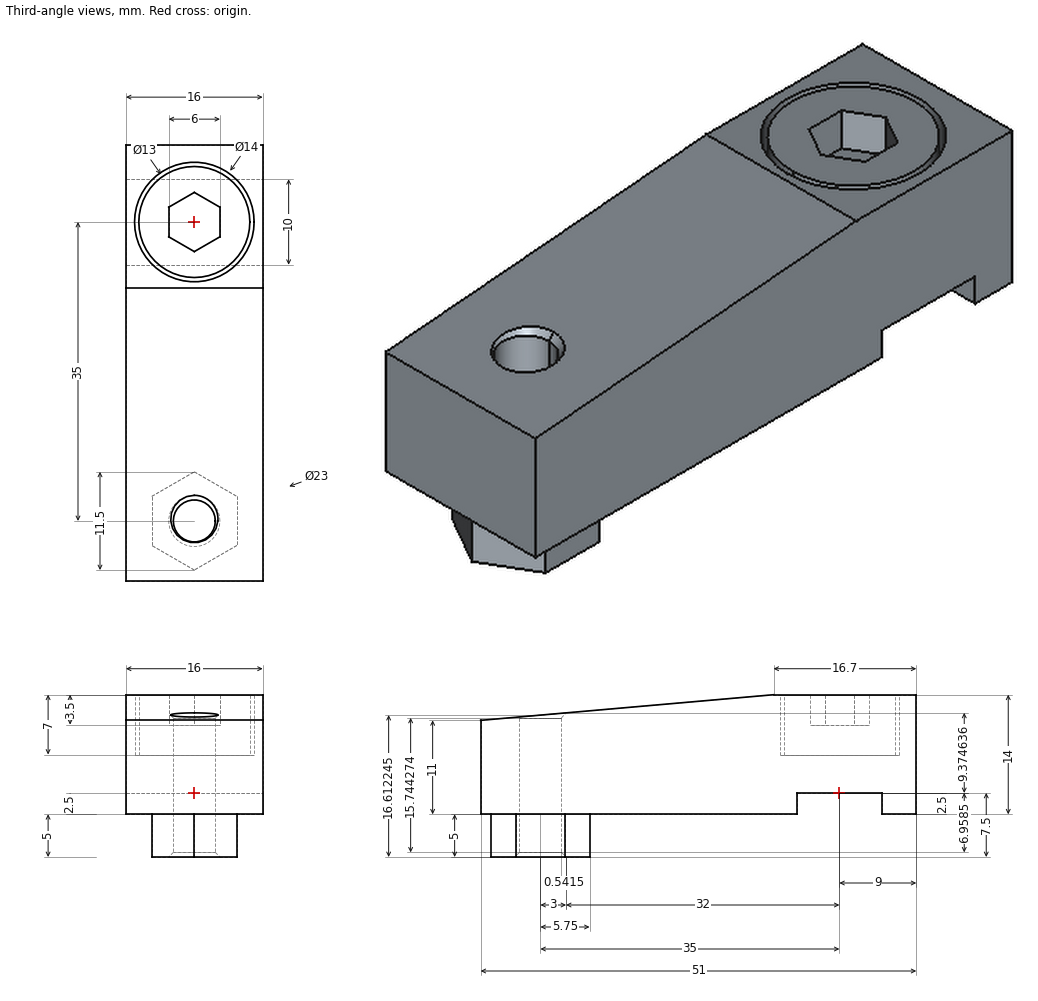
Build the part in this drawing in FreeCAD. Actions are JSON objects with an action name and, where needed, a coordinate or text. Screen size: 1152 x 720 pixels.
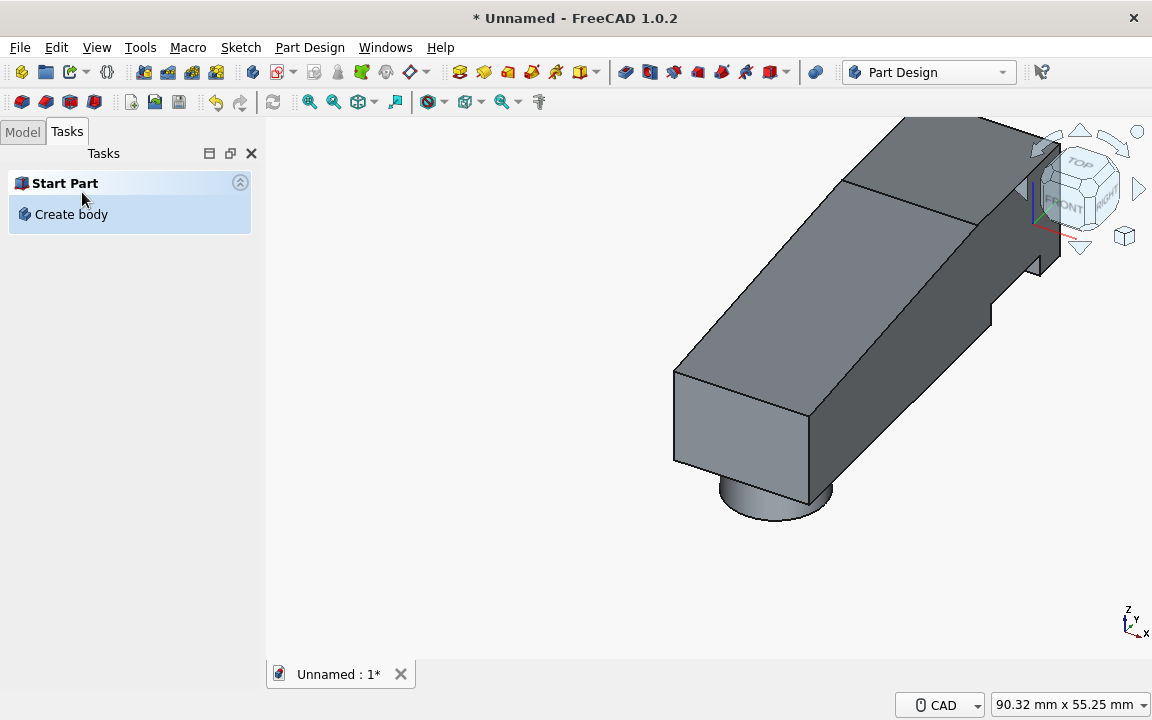
{"action": "left_click", "coordinate": [310, 102]}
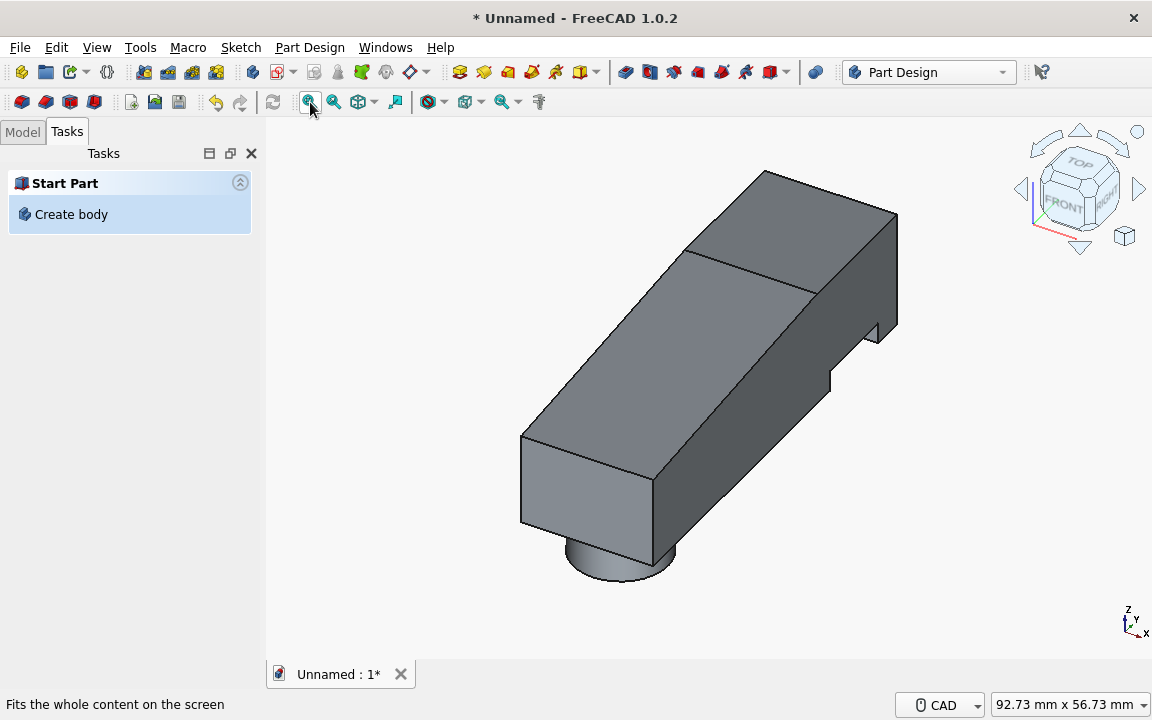
{"action": "key", "text": "5"}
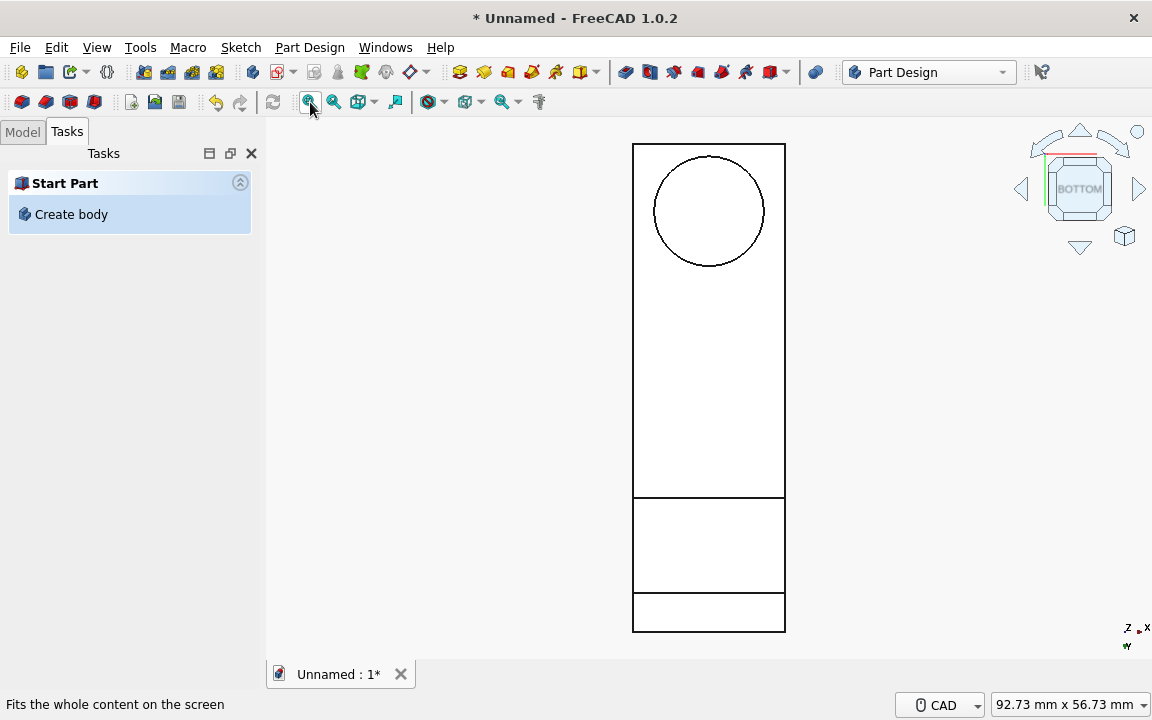
{"action": "left_click", "coordinate": [709, 210]}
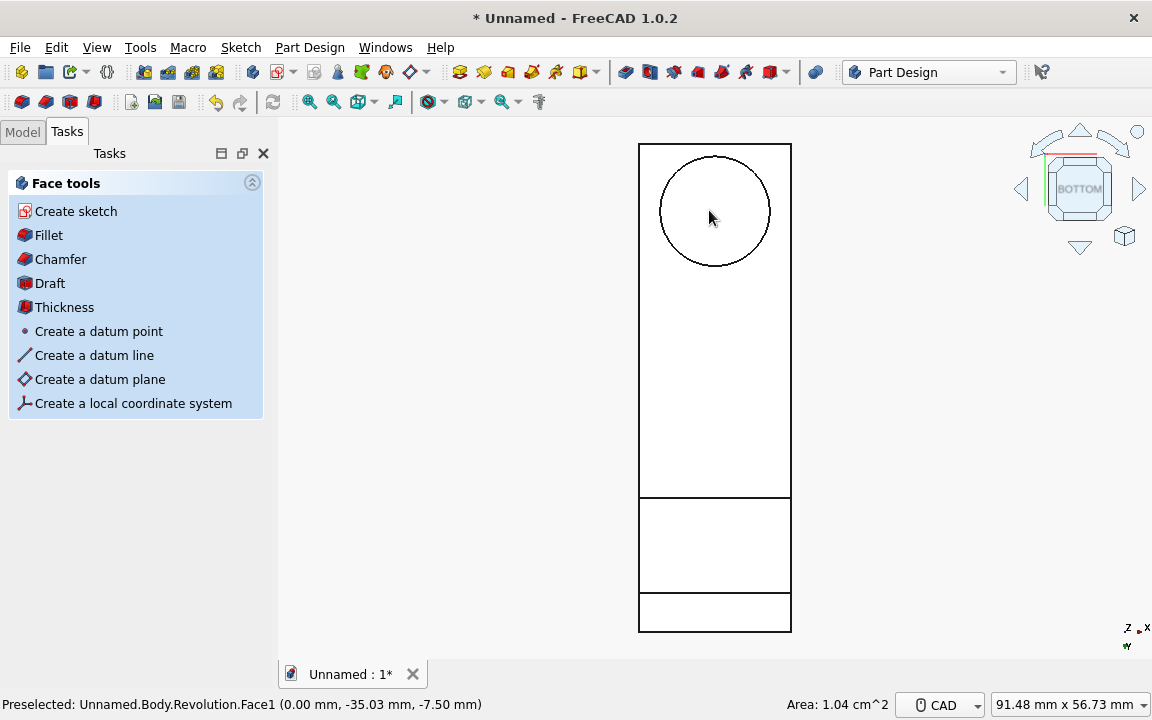
{"action": "left_click", "coordinate": [278, 72]}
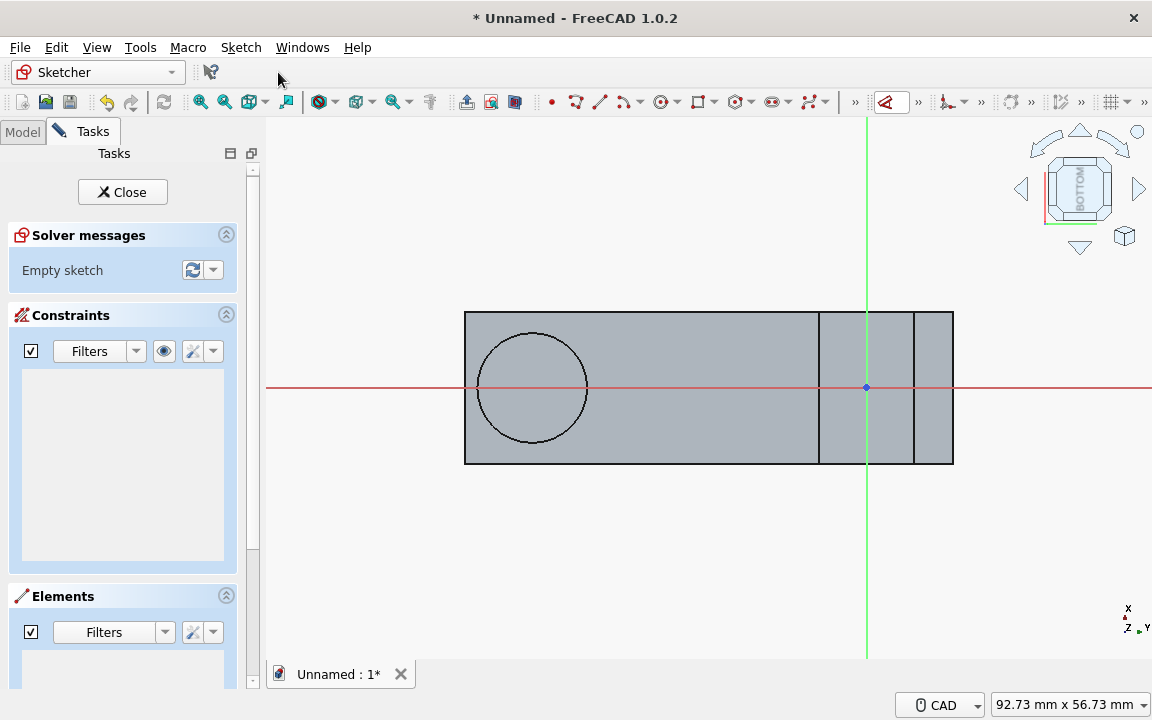
{"action": "left_click", "coordinate": [736, 102]}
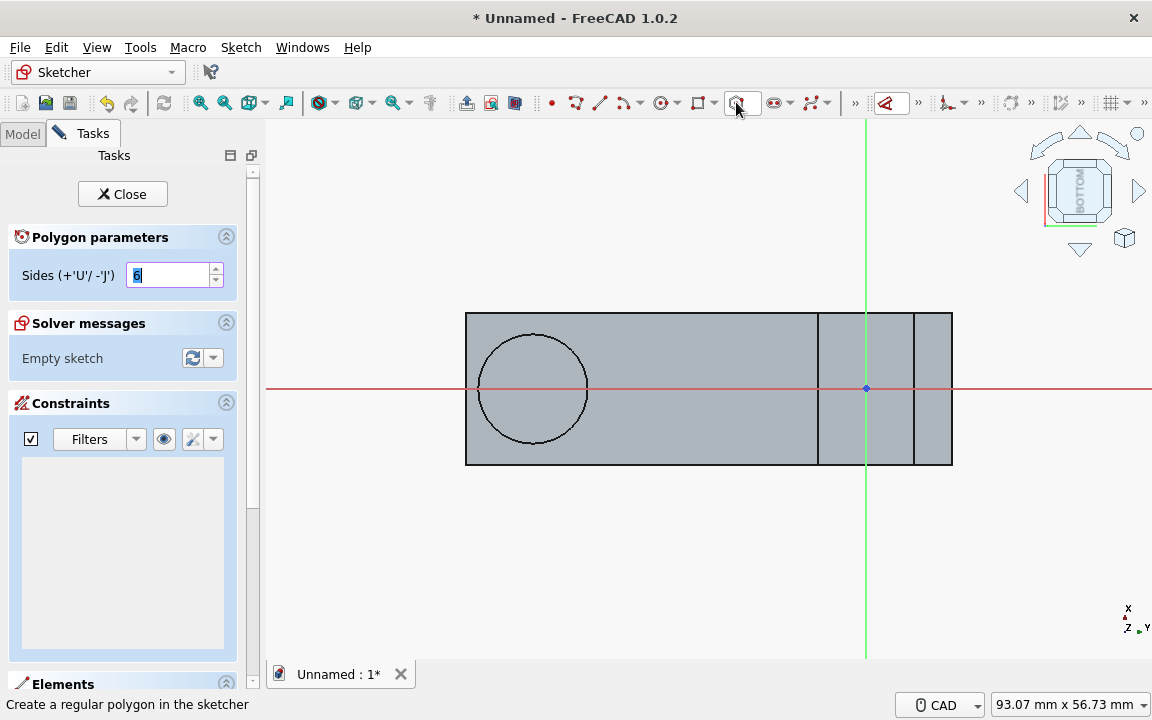
{"action": "left_click", "coordinate": [533, 389]}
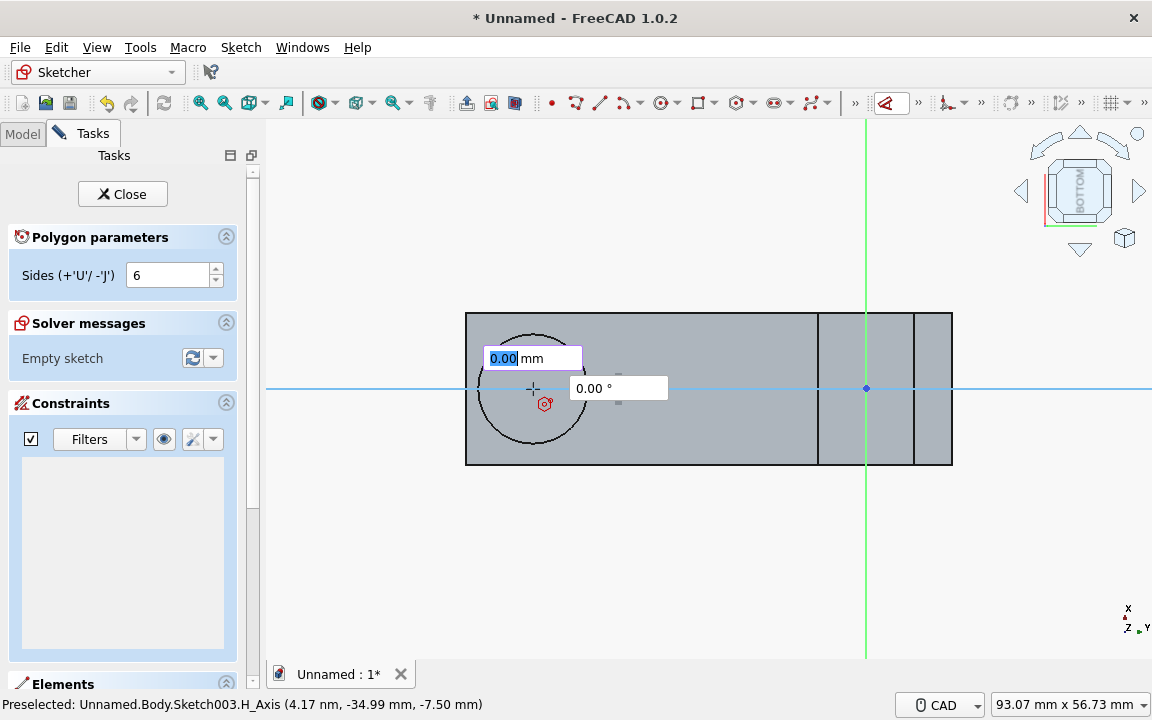
{"action": "left_click", "coordinate": [478, 389]}
{"action": "right_click", "coordinate": [478, 389]}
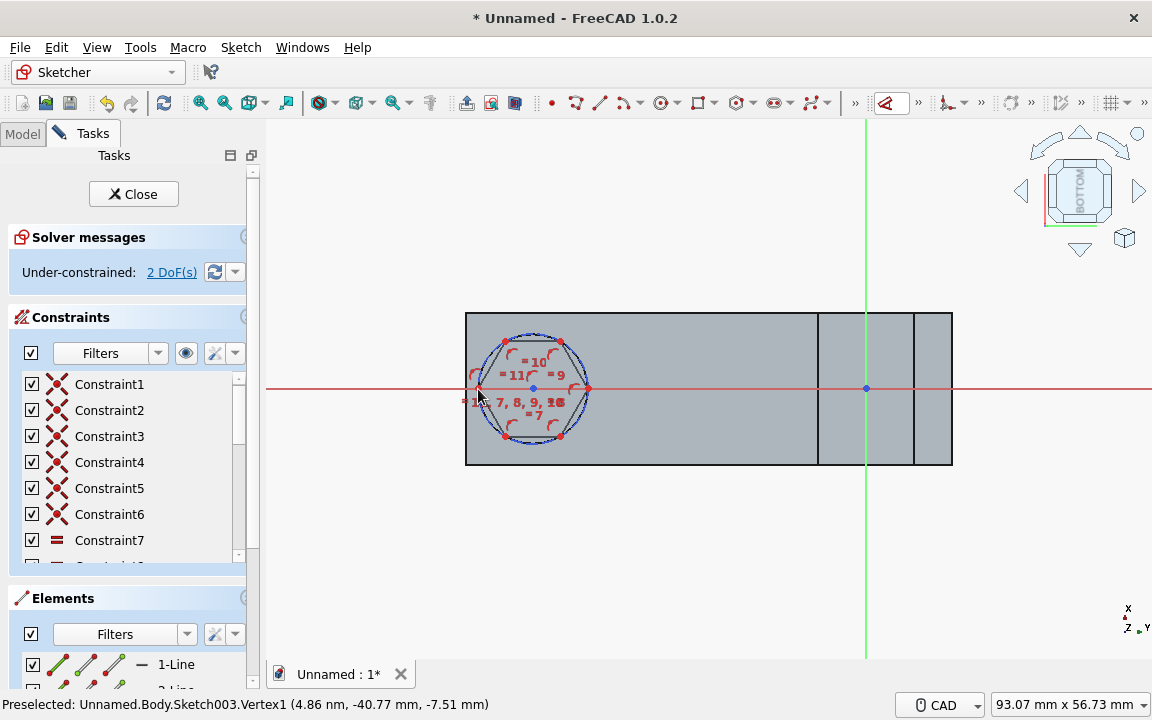
{"action": "left_click", "coordinate": [662, 104]}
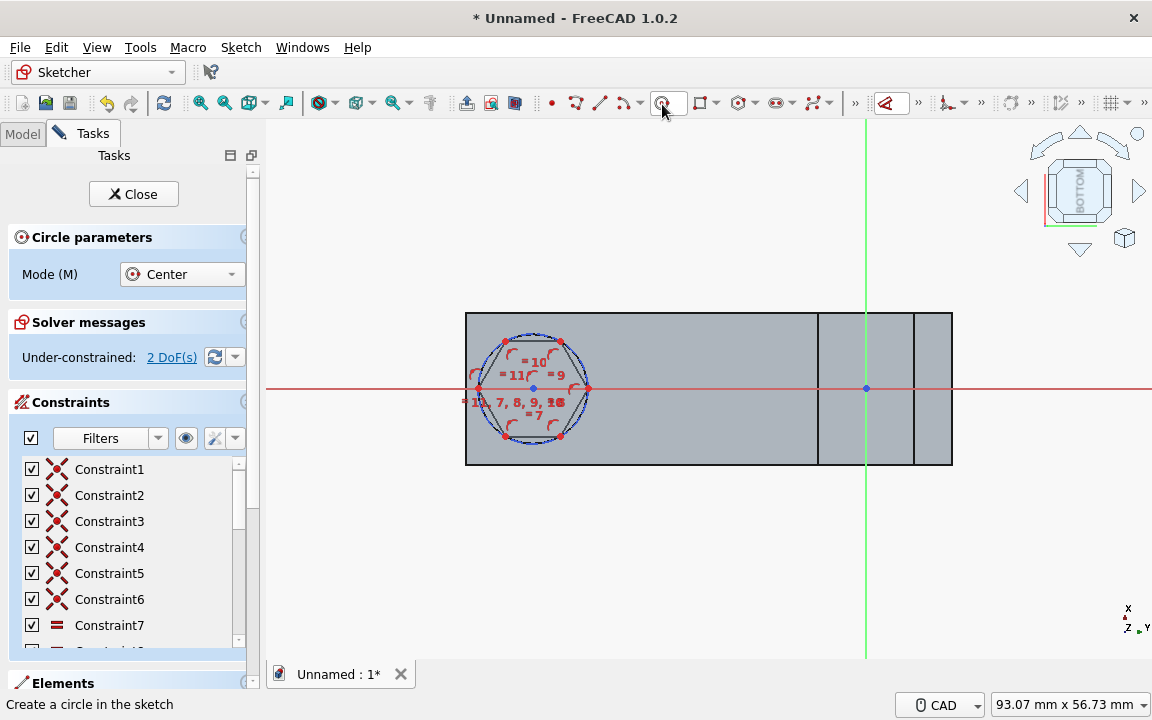
{"action": "left_click", "coordinate": [533, 389]}
{"action": "left_click", "coordinate": [610, 312]}
{"action": "key", "text": "Escape"}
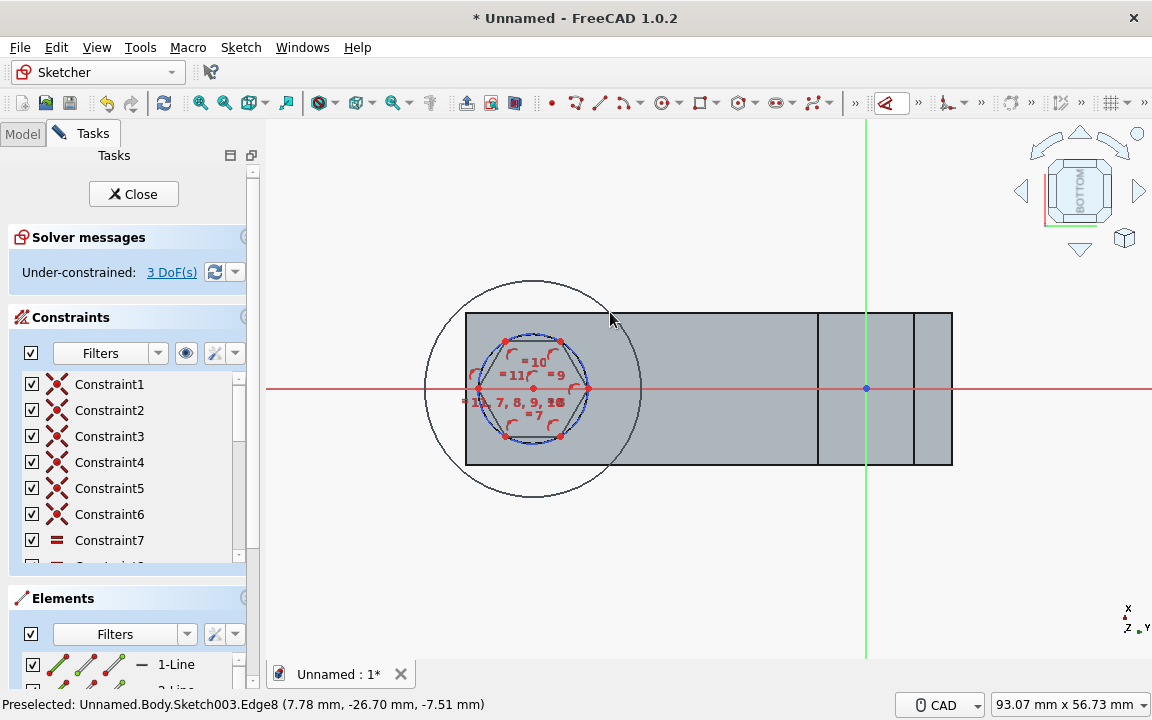
{"action": "left_click", "coordinate": [609, 312]}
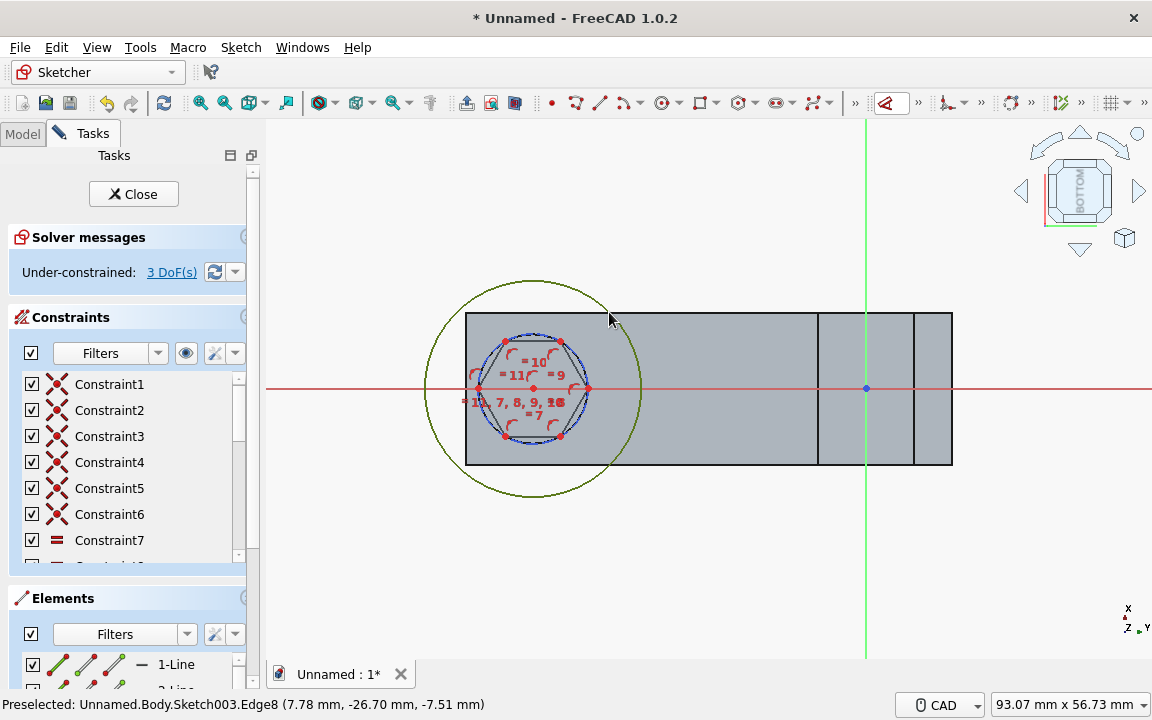
{"action": "left_click", "coordinate": [904, 104]}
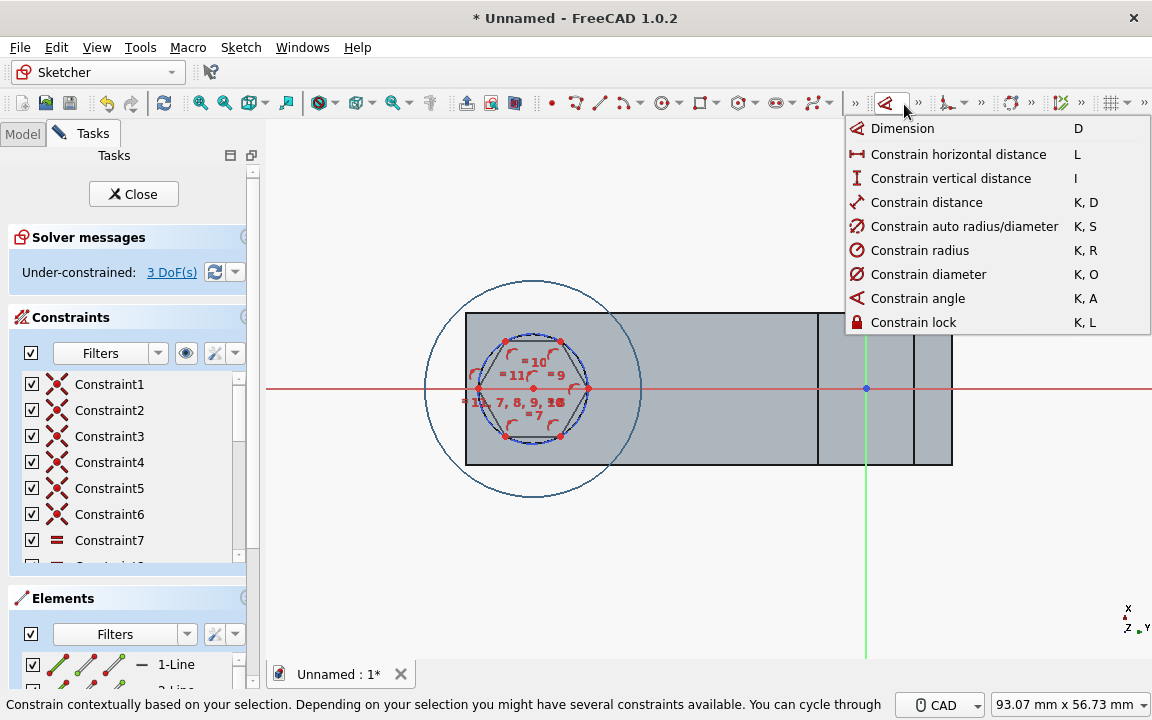
{"action": "left_click", "coordinate": [998, 274]}